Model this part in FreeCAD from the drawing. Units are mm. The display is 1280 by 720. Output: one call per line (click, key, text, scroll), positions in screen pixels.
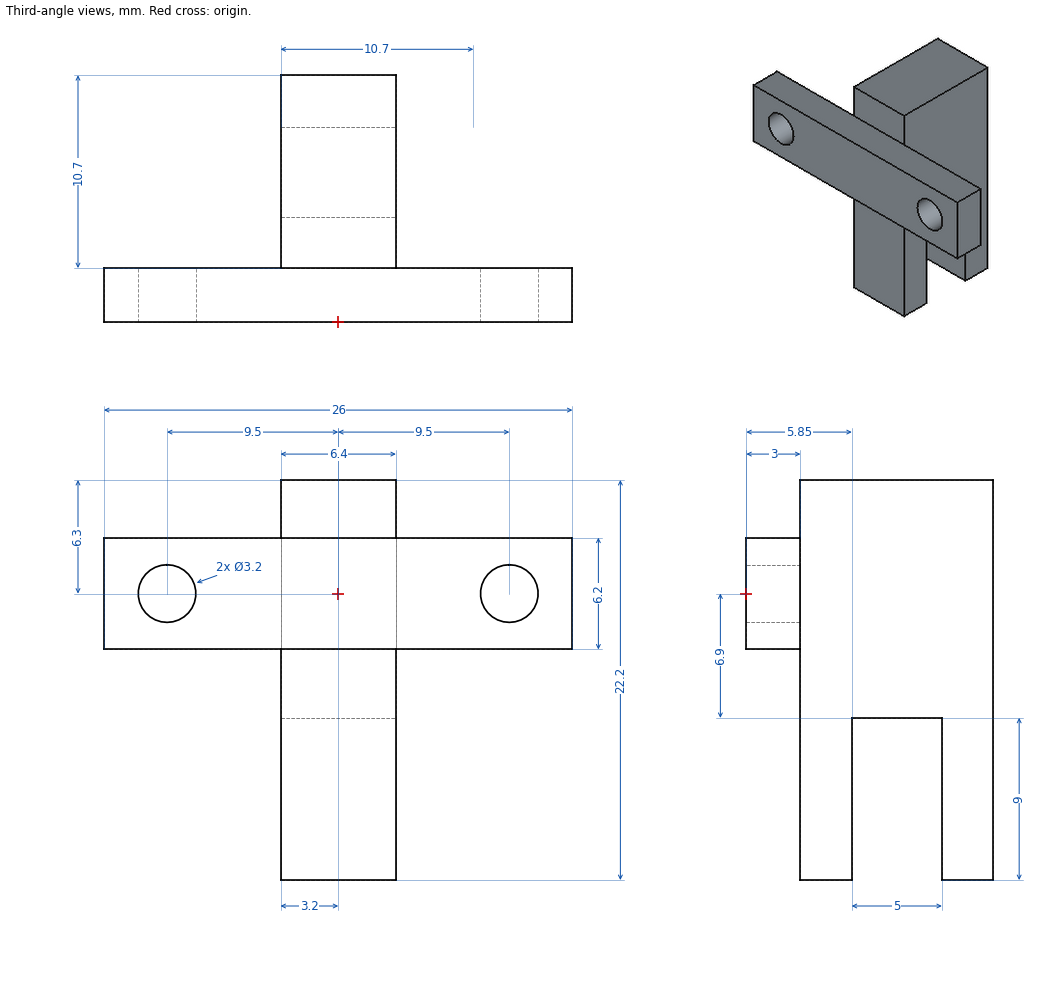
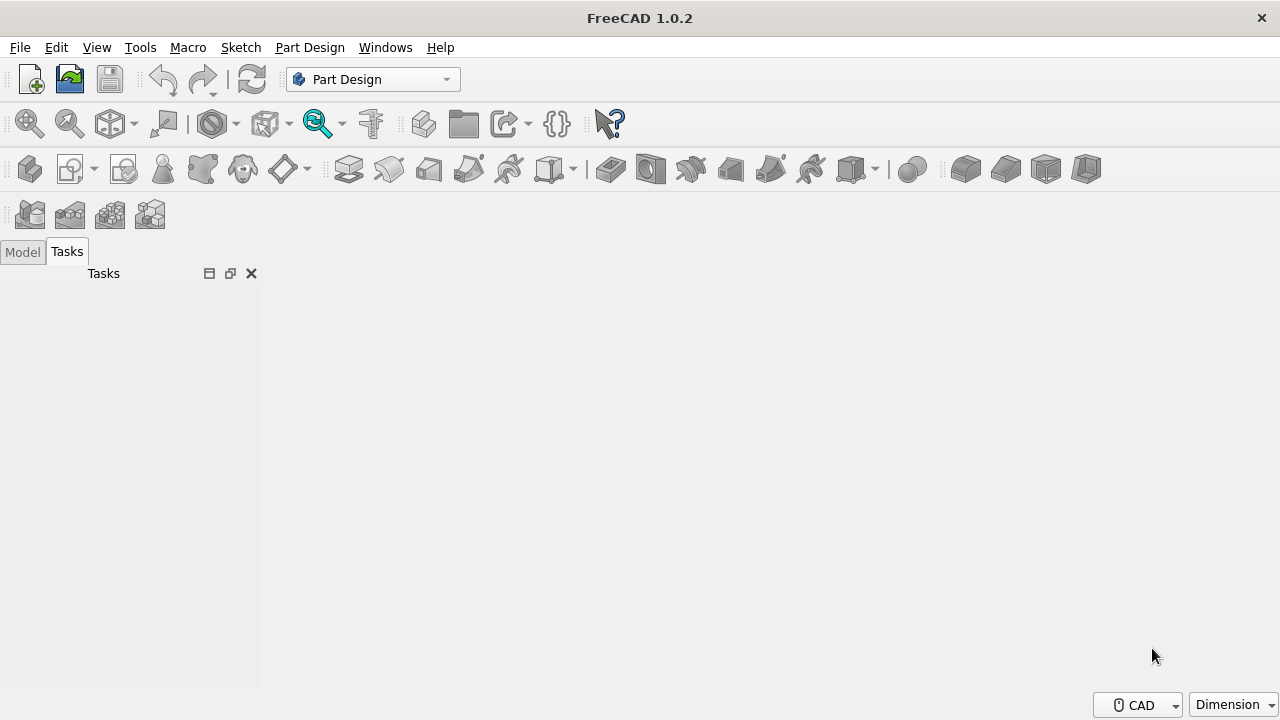
click(30, 80)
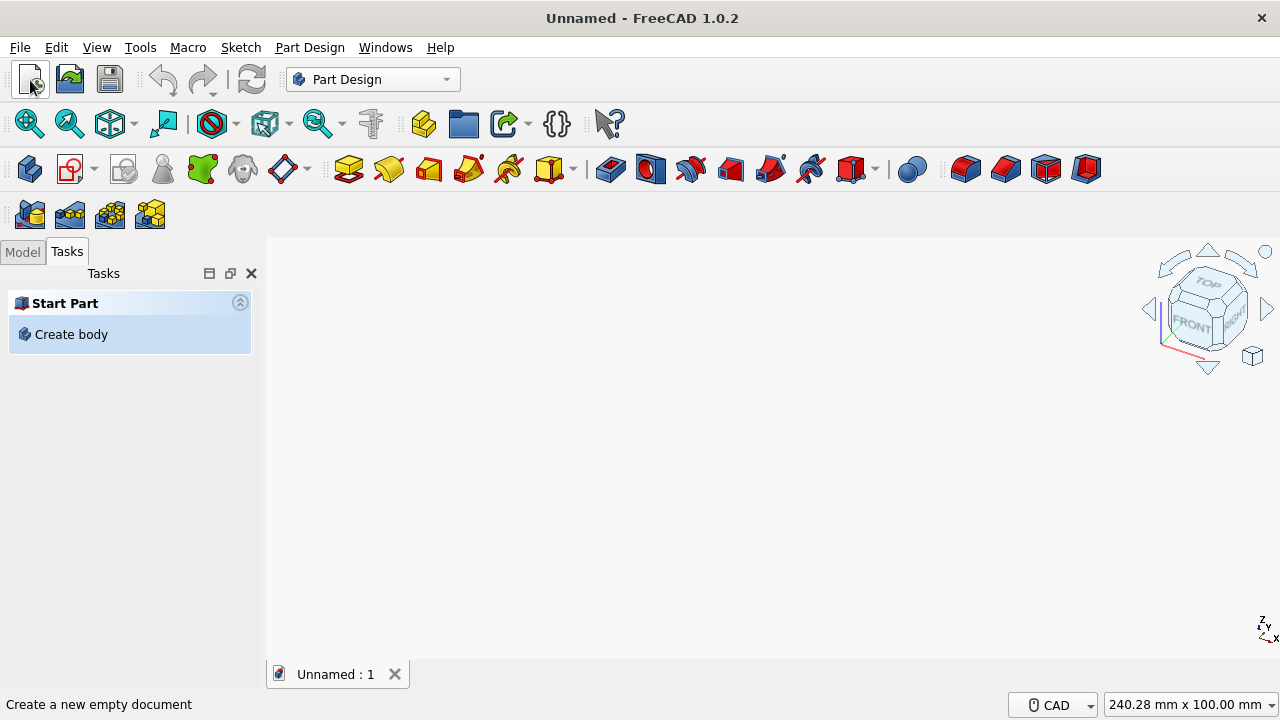
click(70, 170)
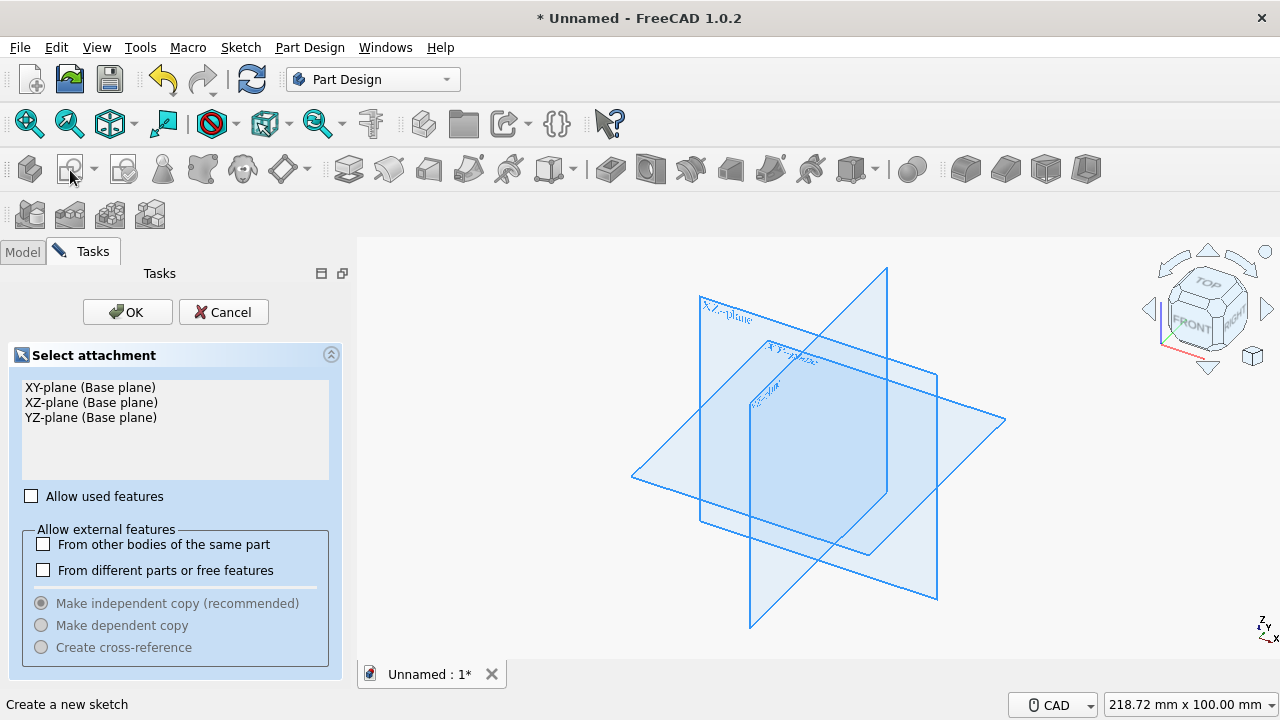
click(82, 402)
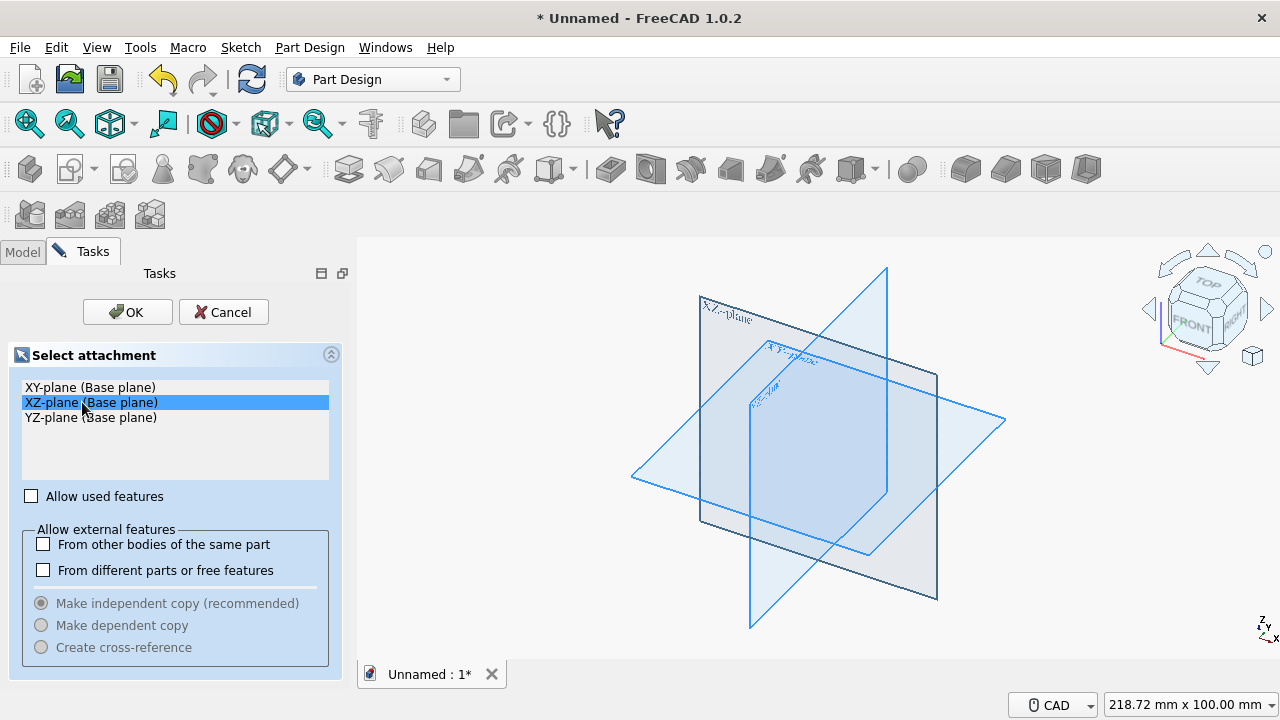
click(128, 312)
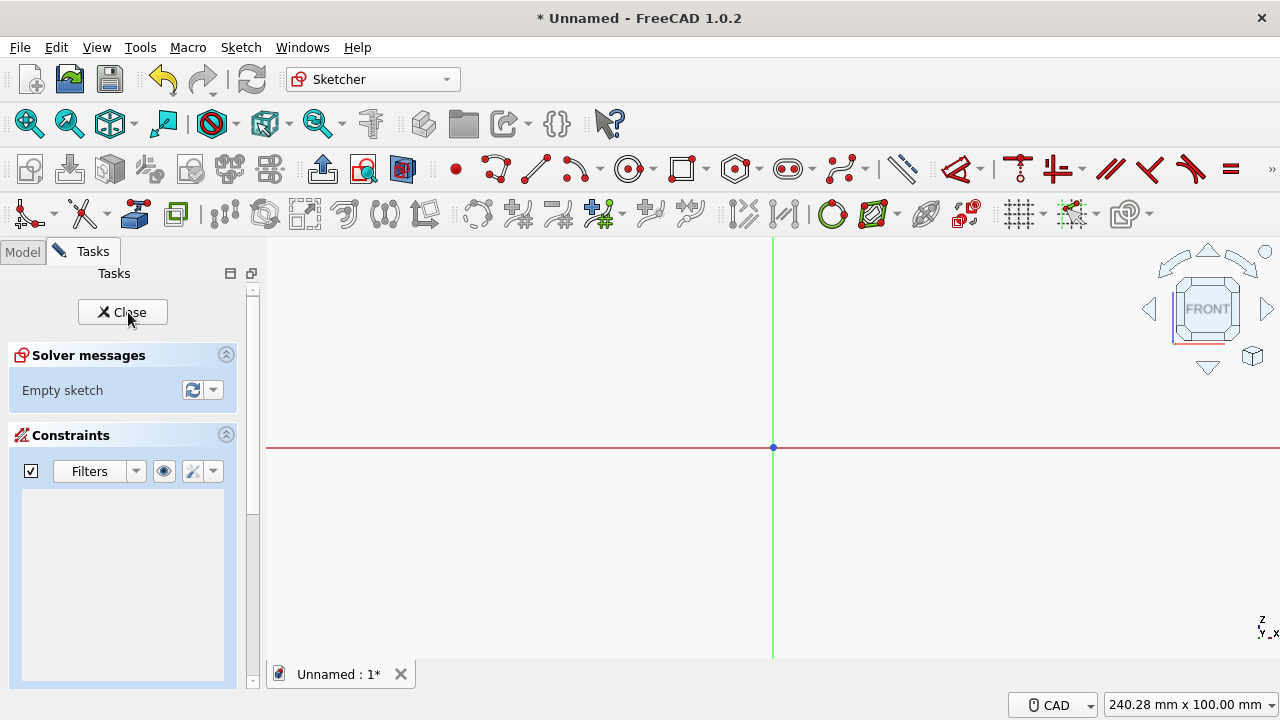
scroll(790, 448, up, 8)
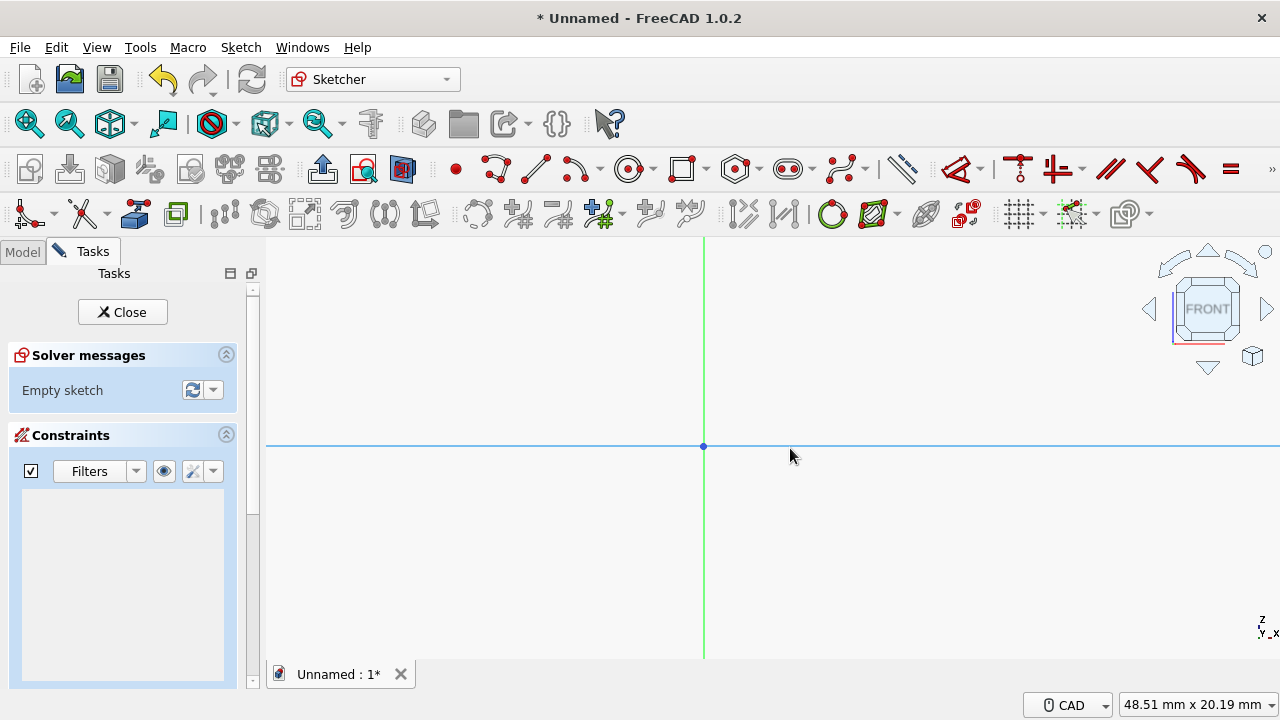
key(g)
key(v)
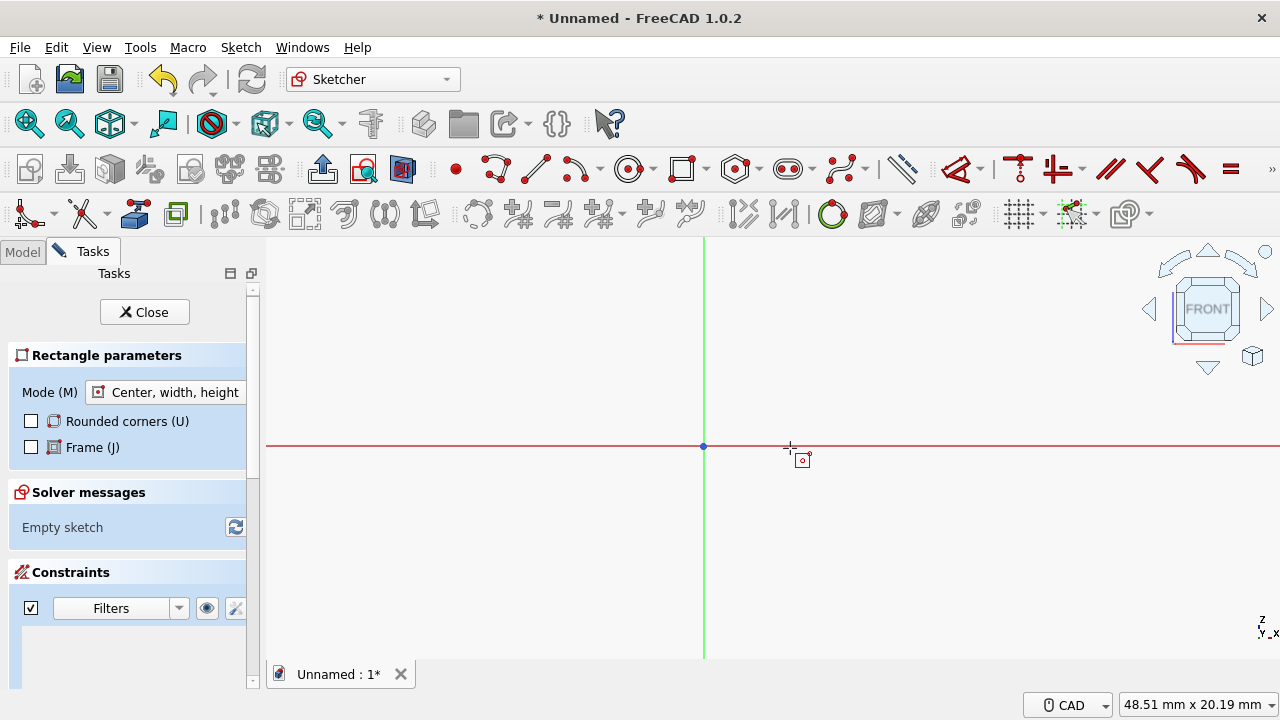
click(704, 446)
move(975, 381)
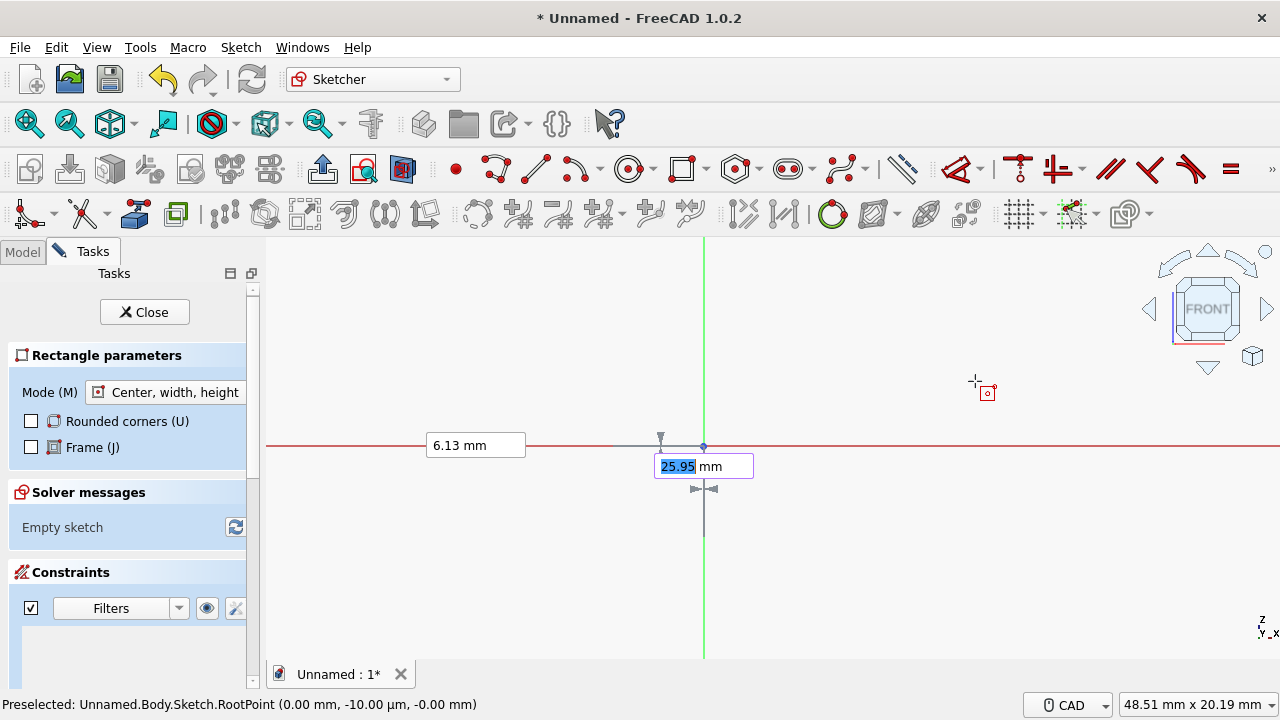
text(26)
key(Tab)
text(6.2)
key(Return)
key(Escape)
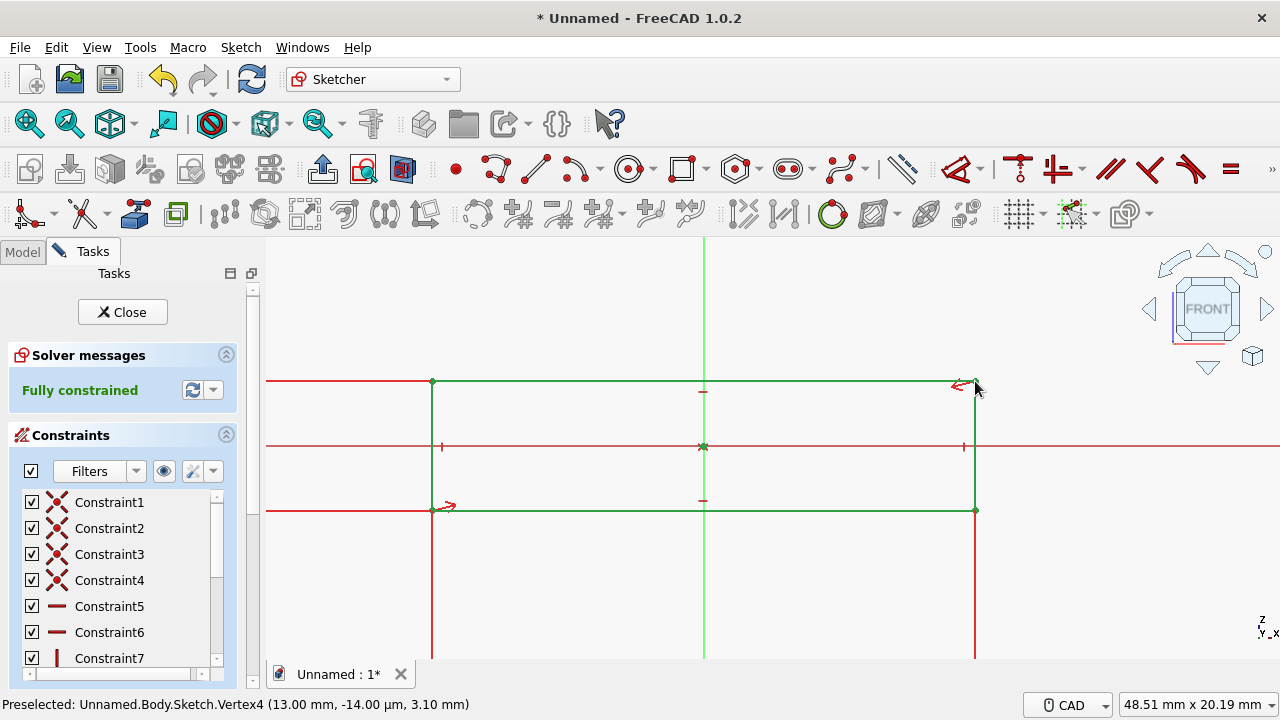
click(123, 312)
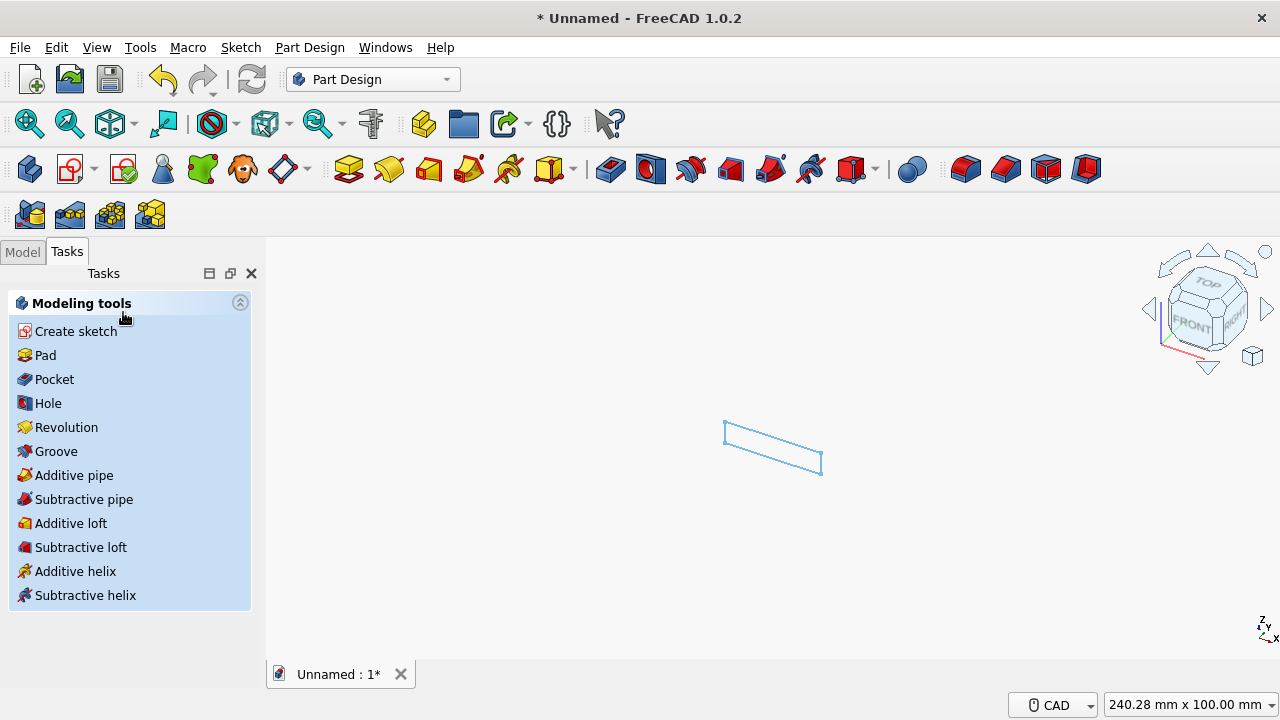
click(350, 170)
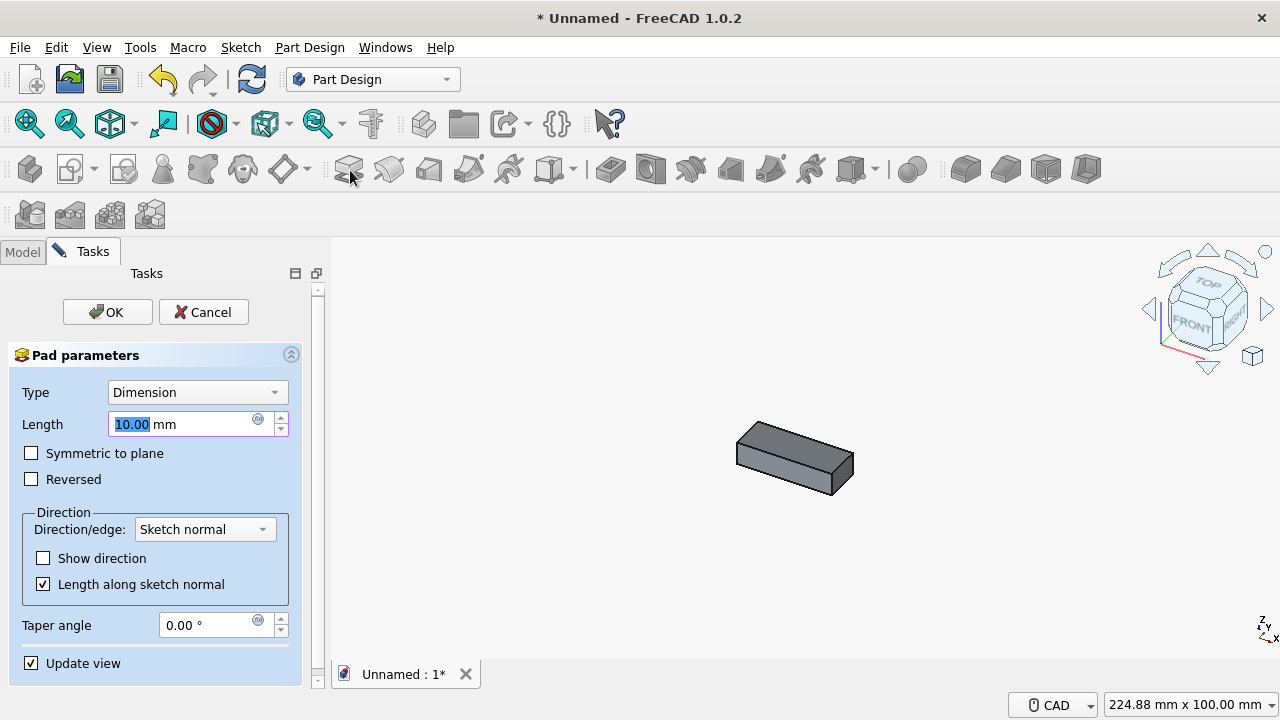
text(3)
key(Tab)